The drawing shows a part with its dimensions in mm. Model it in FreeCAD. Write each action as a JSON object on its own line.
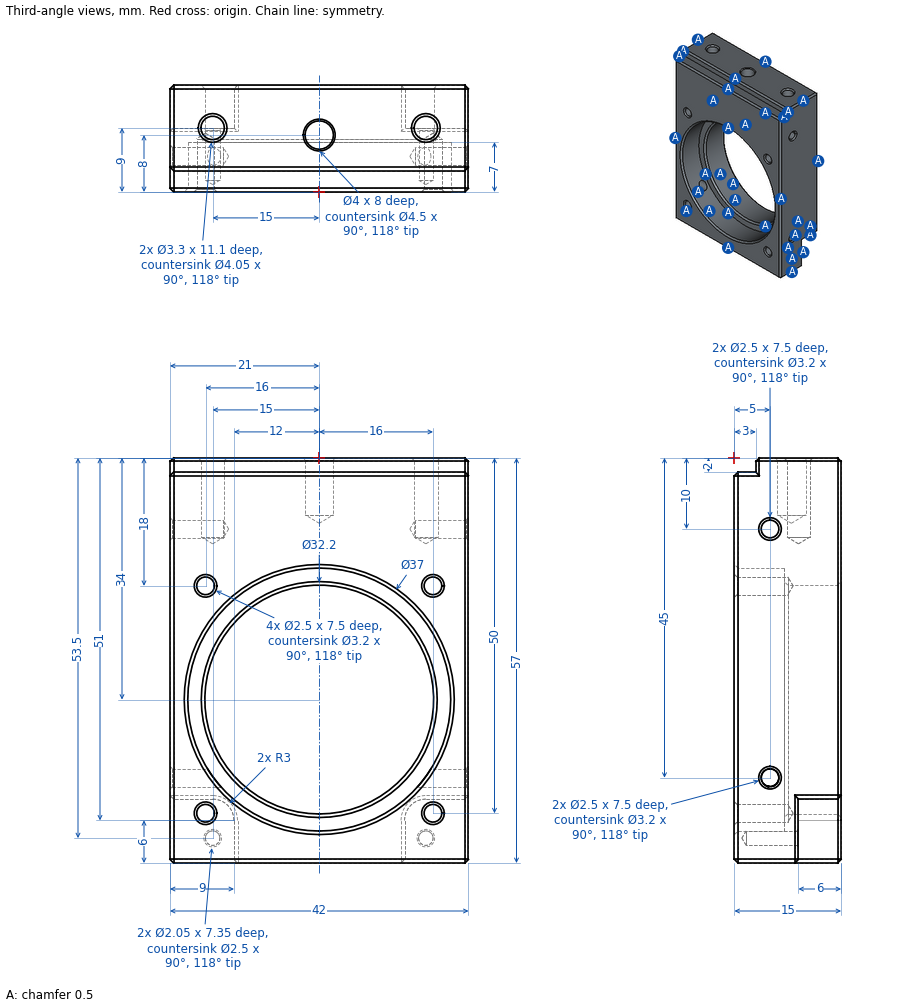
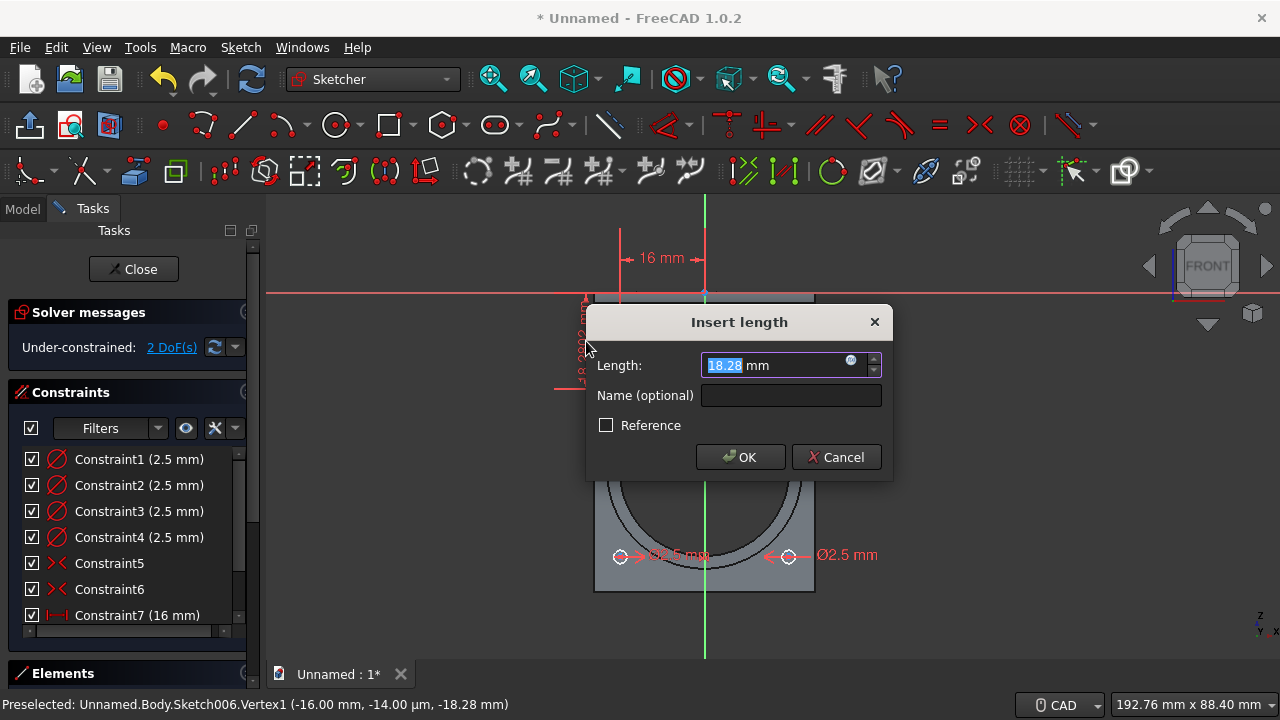
{"action": "type", "text": "18"}
{"action": "key", "text": "Return"}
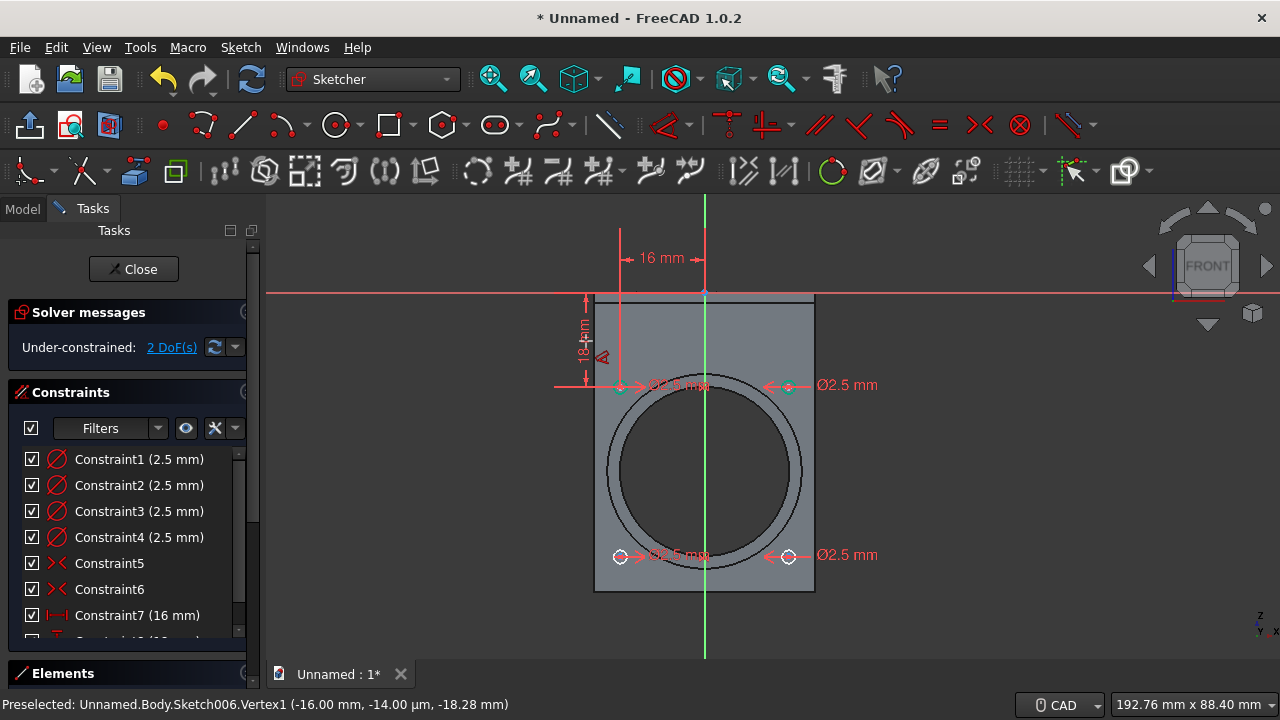
{"action": "left_click", "coordinate": [789, 557]}
{"action": "left_click", "coordinate": [747, 259]}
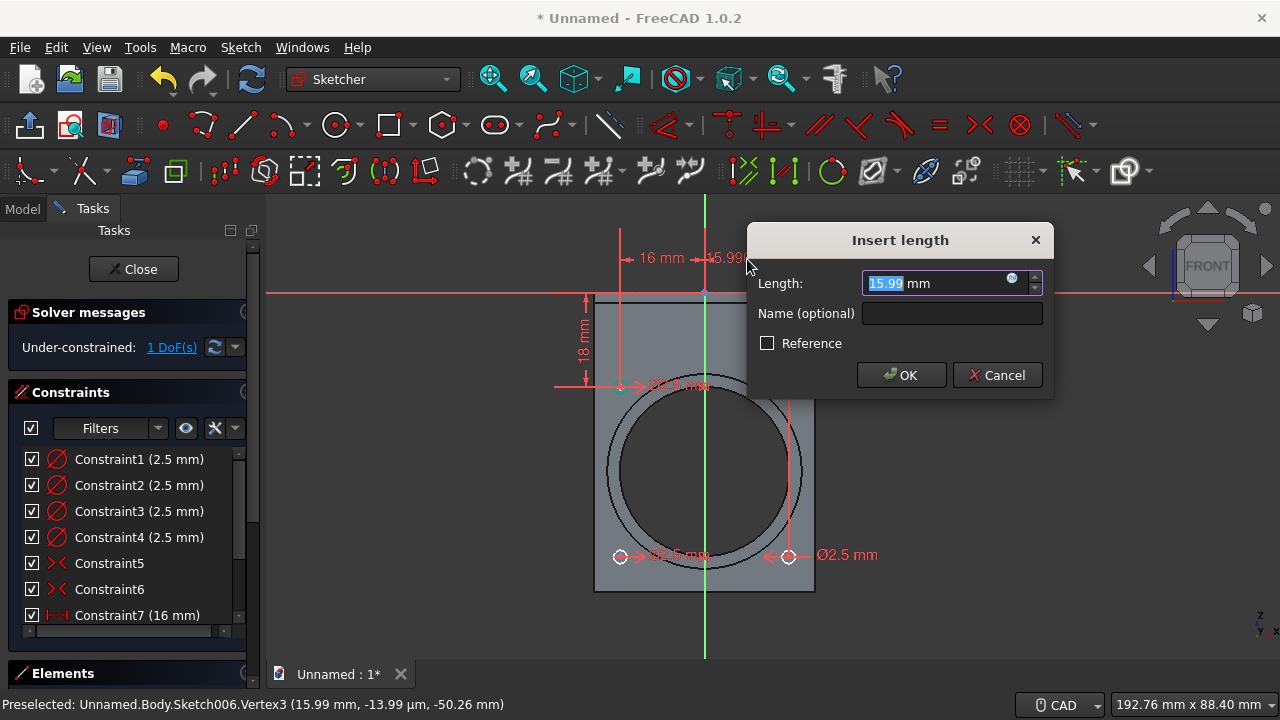
{"action": "type", "text": "16"}
{"action": "key", "text": "Return"}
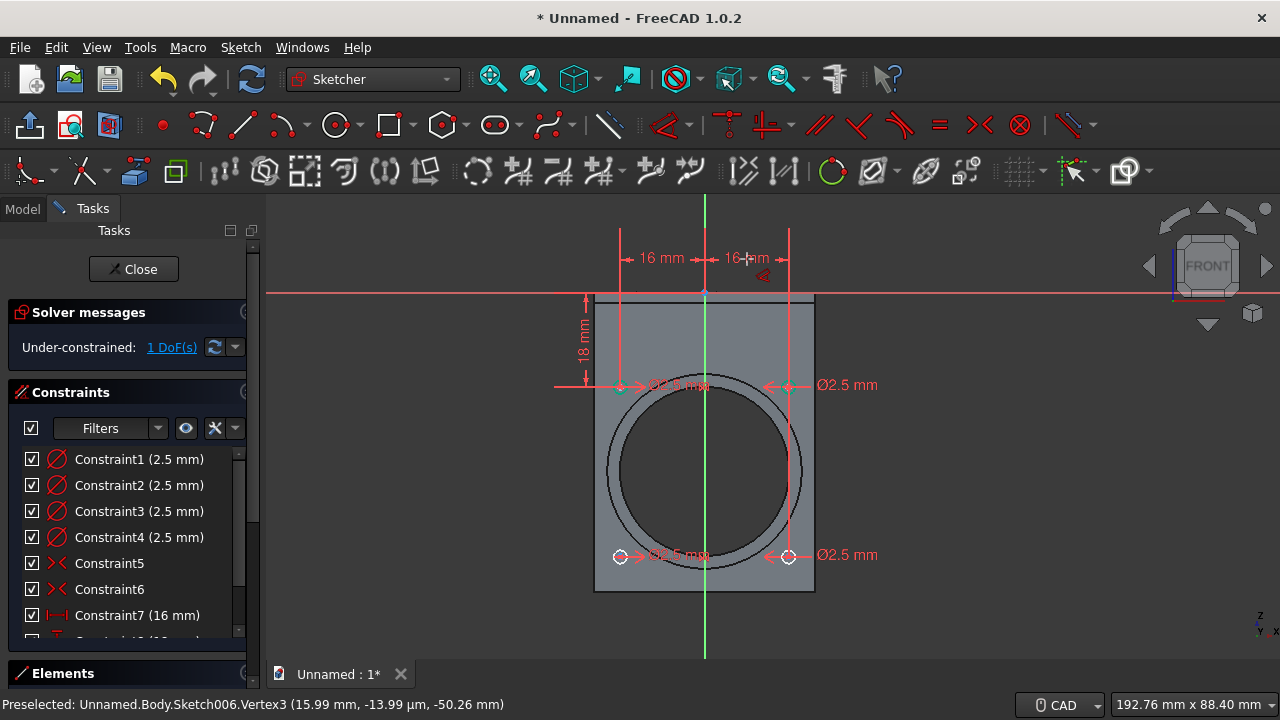
{"action": "left_click", "coordinate": [789, 557]}
{"action": "left_click", "coordinate": [823, 425]}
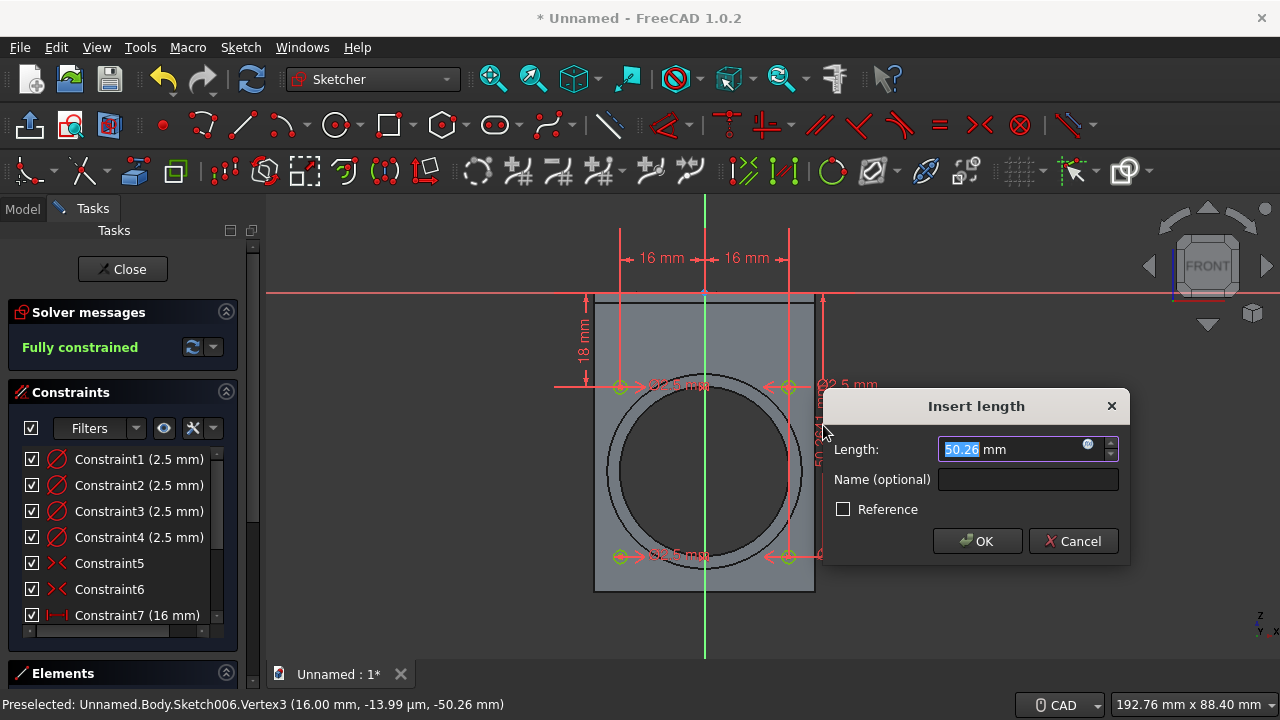
{"action": "type", "text": "50"}
{"action": "key", "text": "Return"}
{"action": "key", "text": "Escape"}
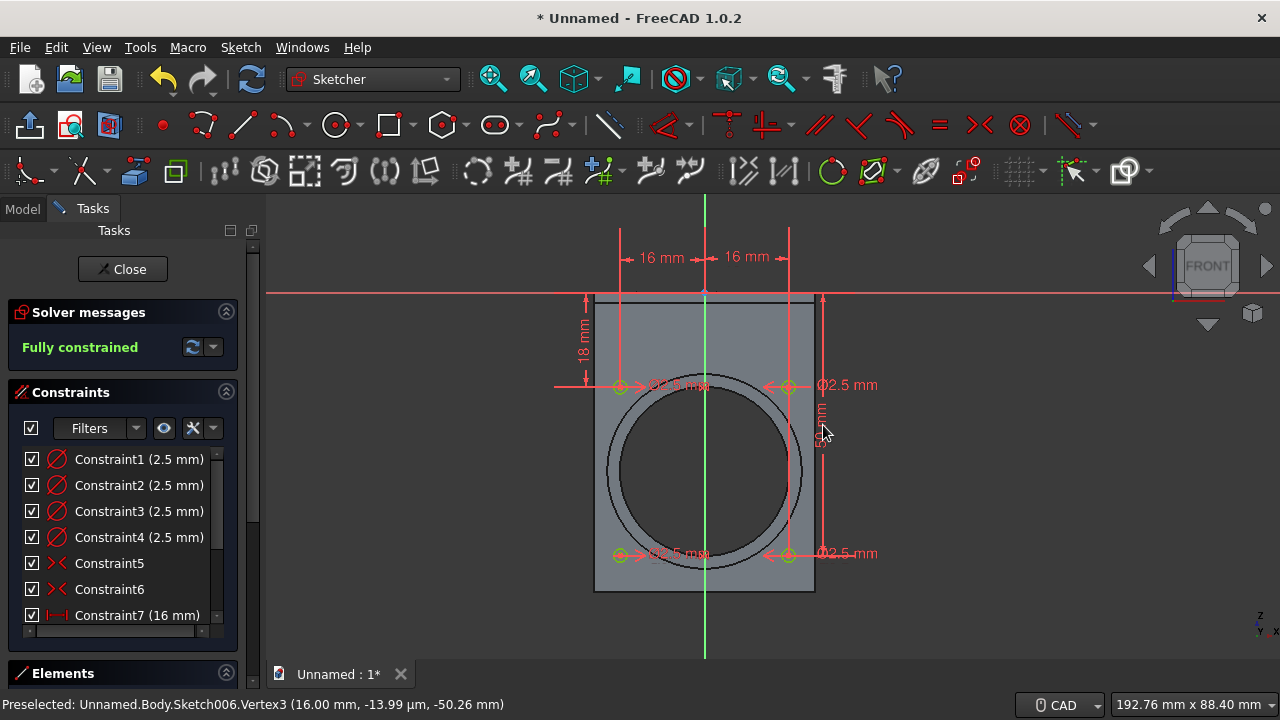
{"action": "left_click", "coordinate": [123, 269]}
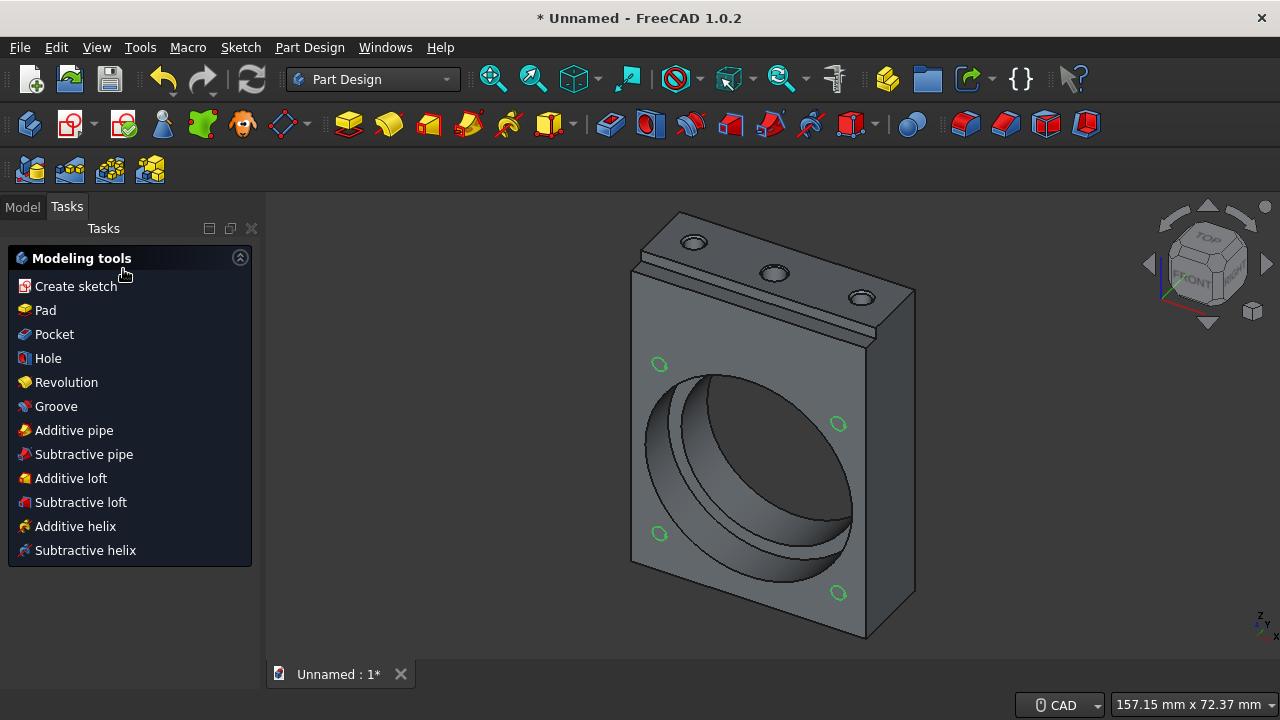
{"action": "left_click", "coordinate": [652, 124]}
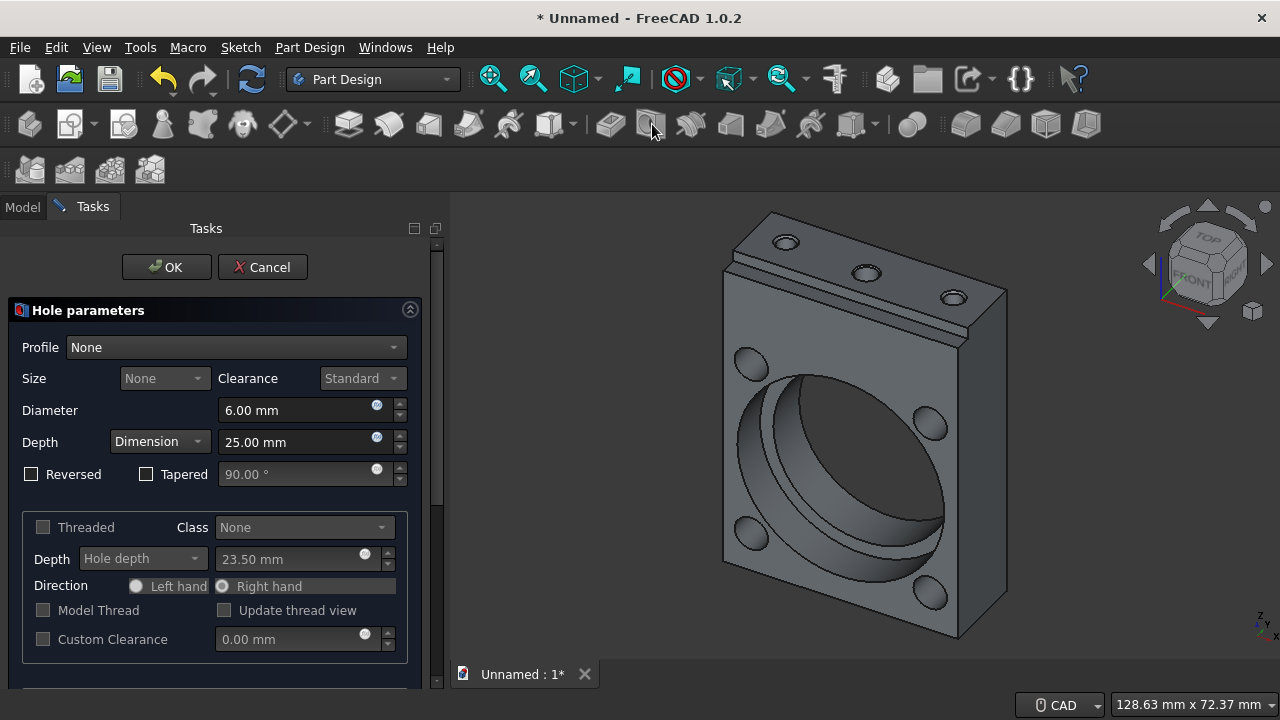
{"action": "triple_click", "coordinate": [305, 410]}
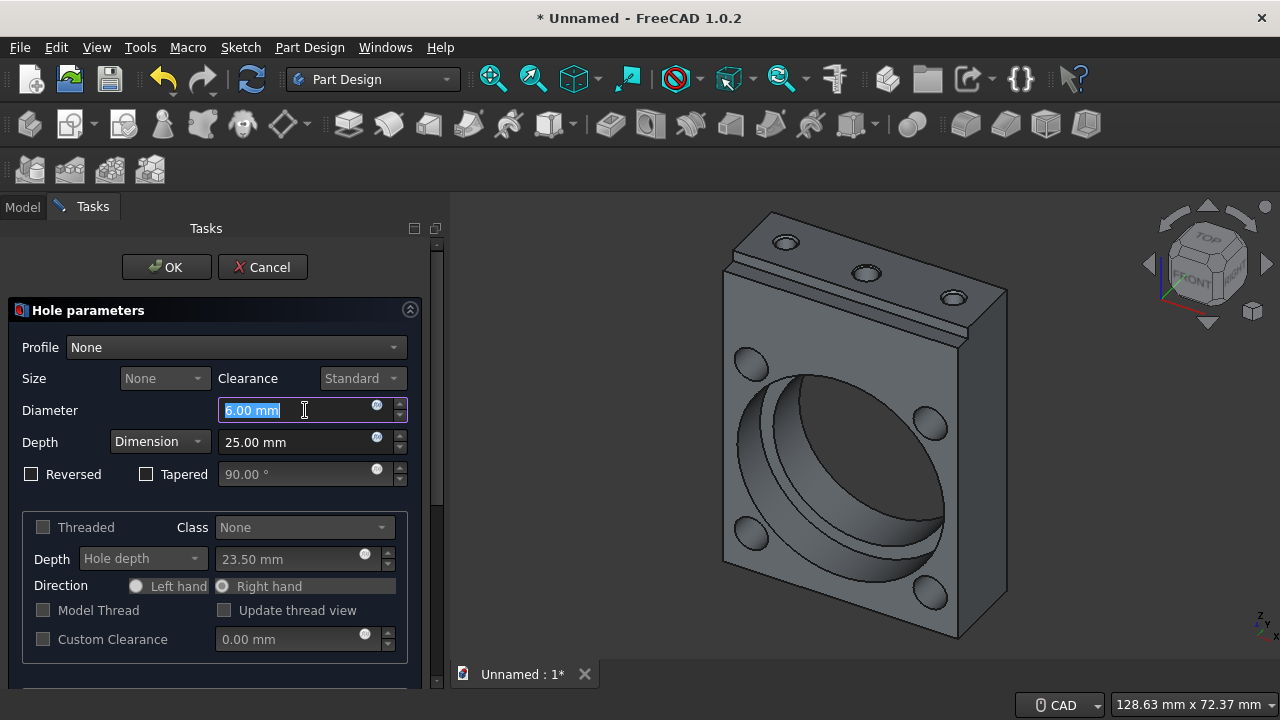
{"action": "type", "text": "2.5"}
{"action": "key", "text": "Tab"}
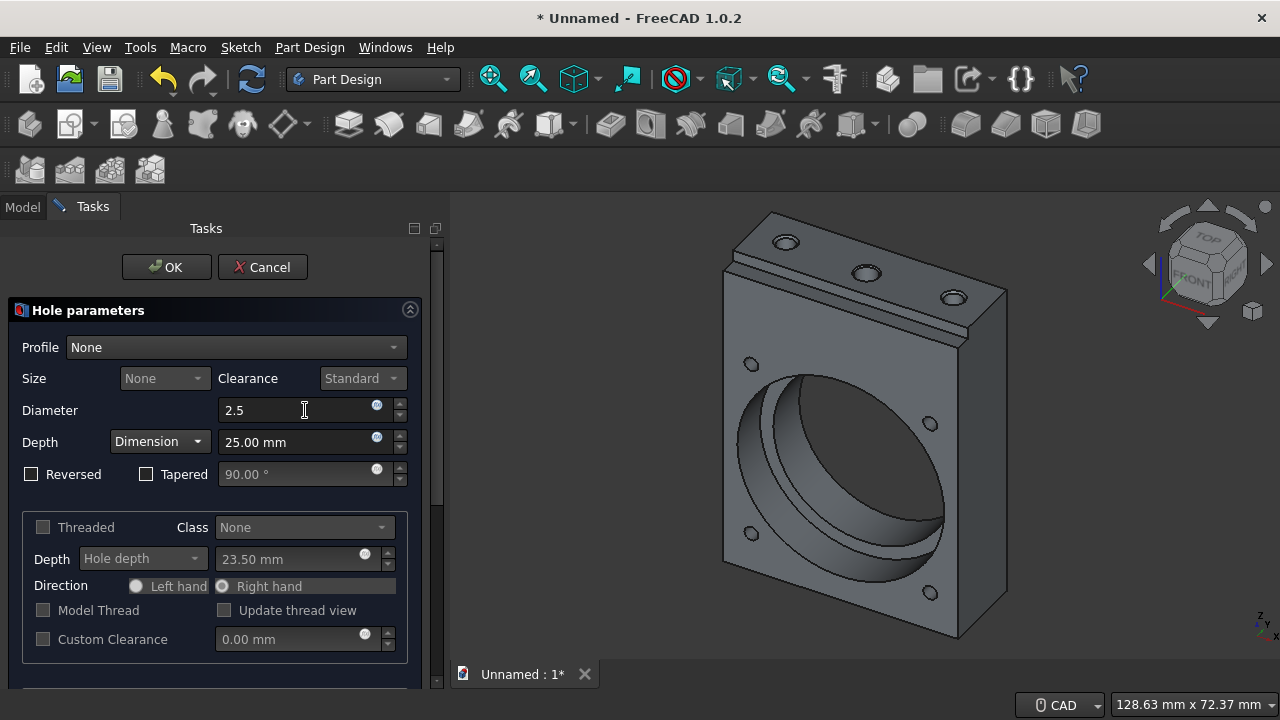
{"action": "triple_click", "coordinate": [305, 442]}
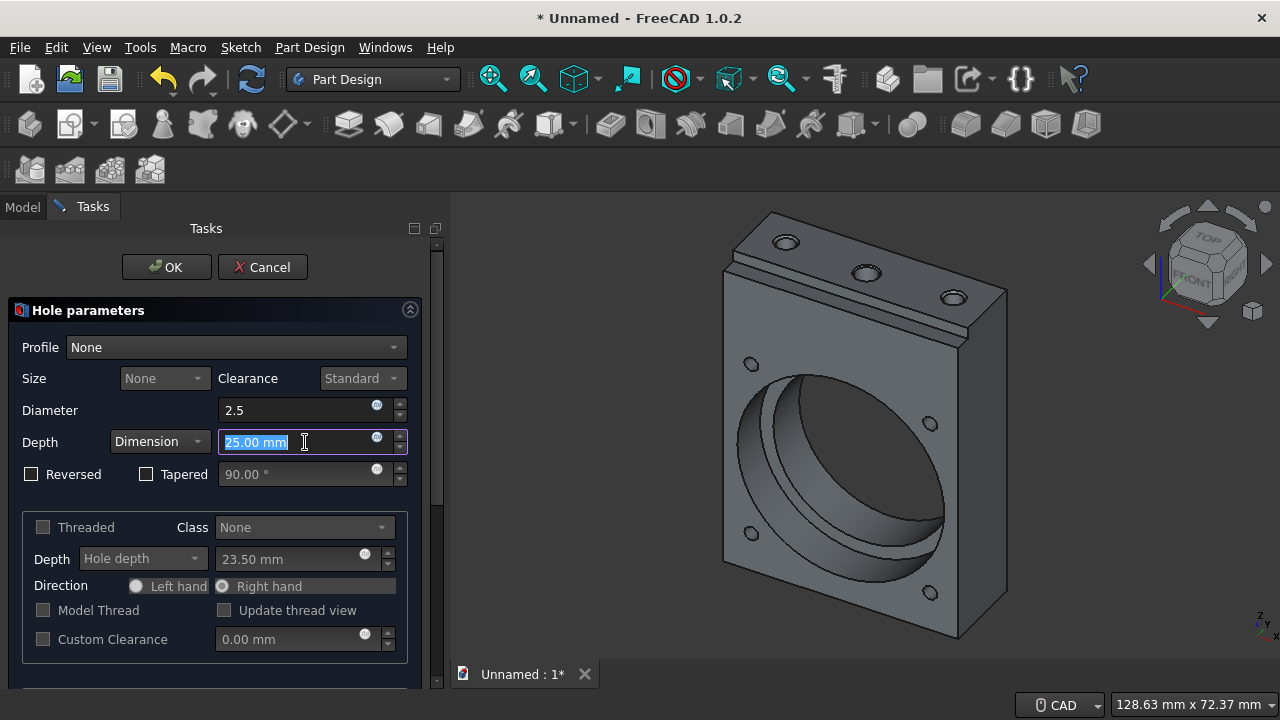
{"action": "type", "text": "7.5"}
{"action": "key", "text": "Tab"}